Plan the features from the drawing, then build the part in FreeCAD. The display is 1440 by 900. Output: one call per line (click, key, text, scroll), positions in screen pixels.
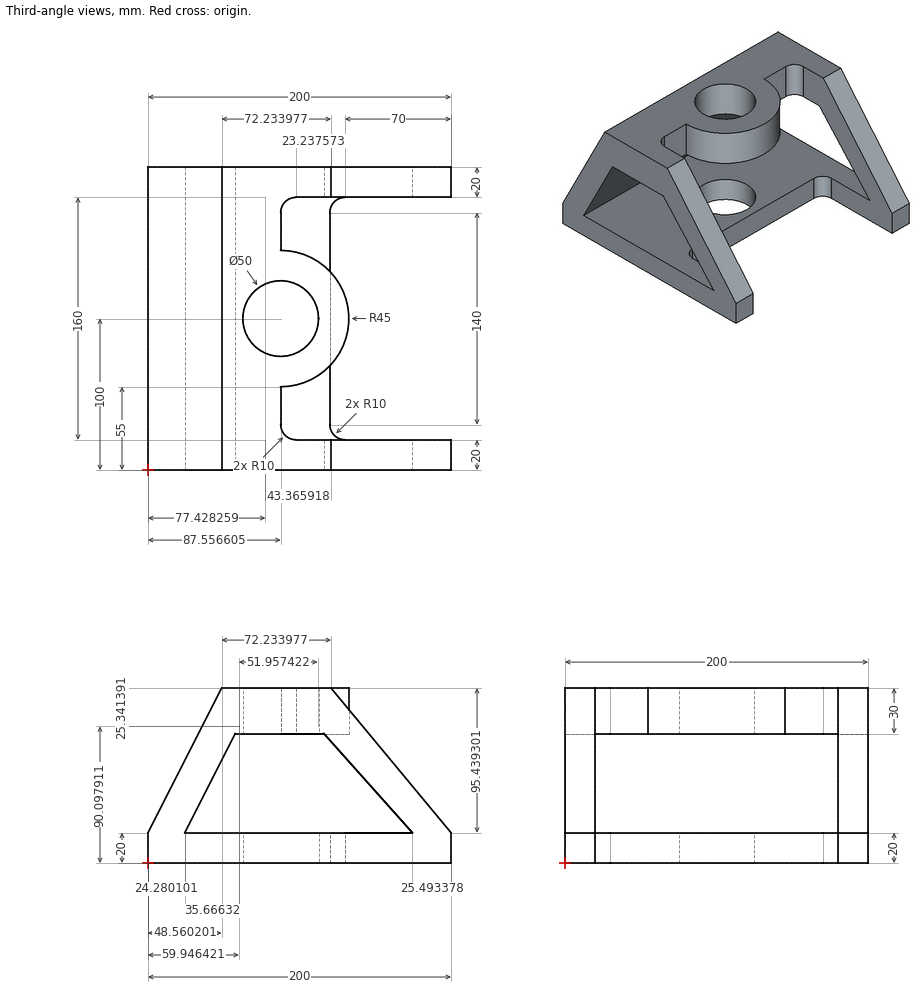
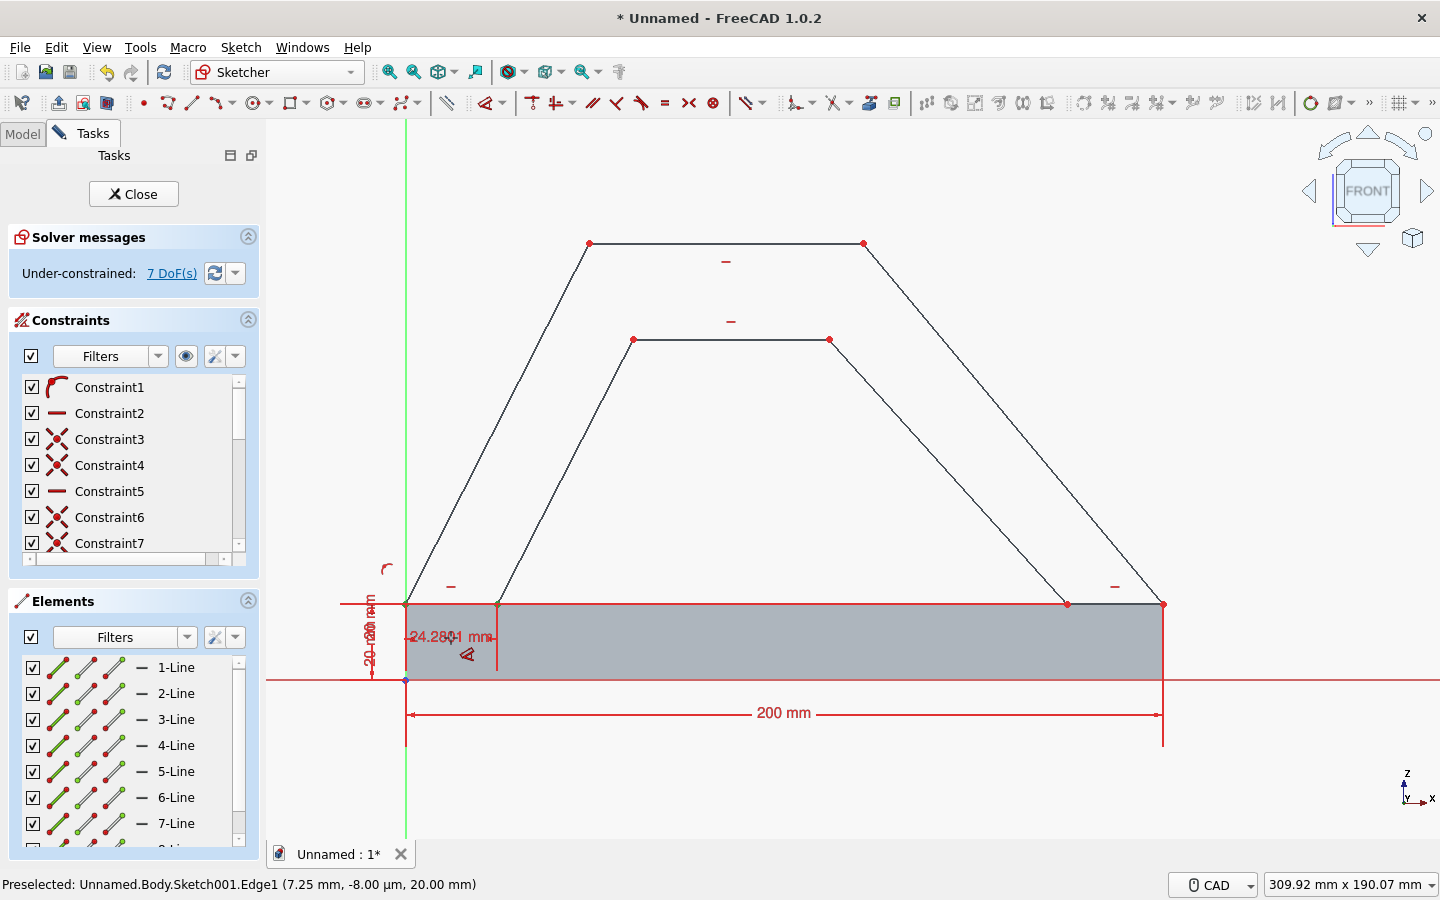
click(692, 340)
click(731, 306)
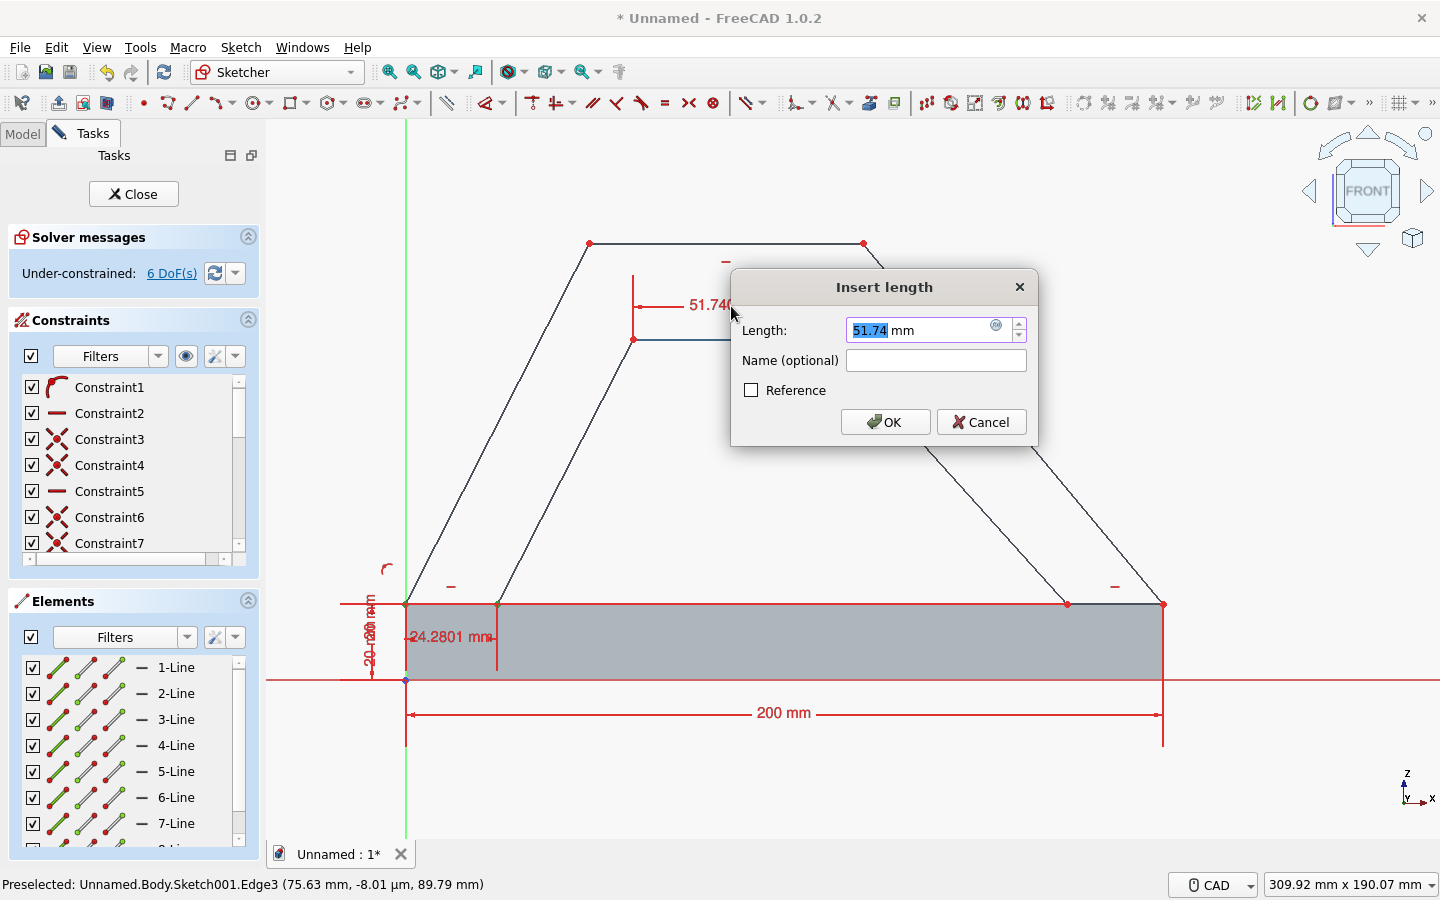
text(51.957422)
key(Return)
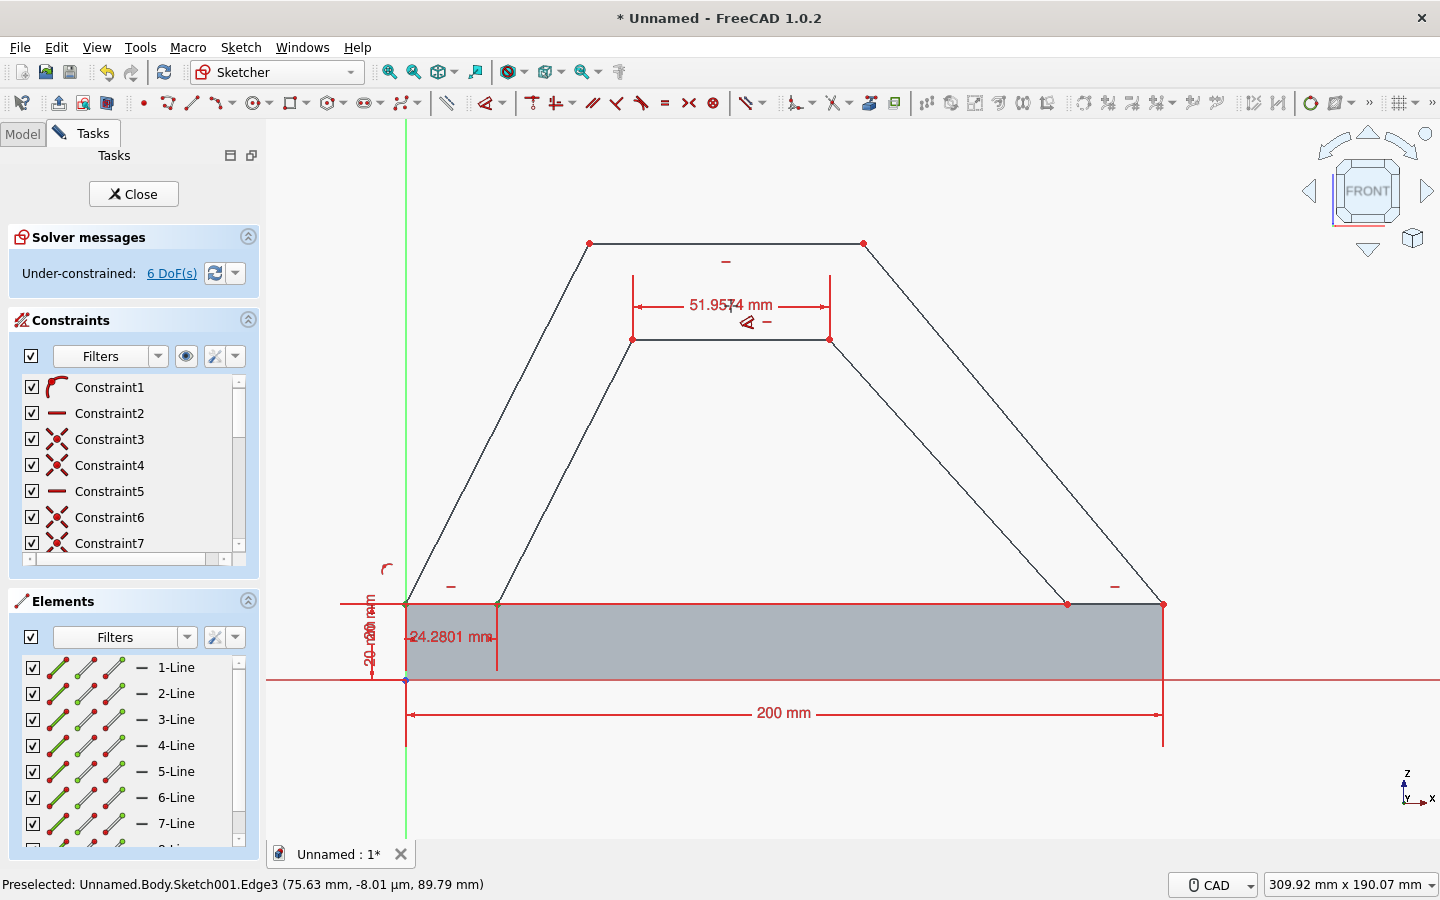
click(1096, 604)
click(1115, 638)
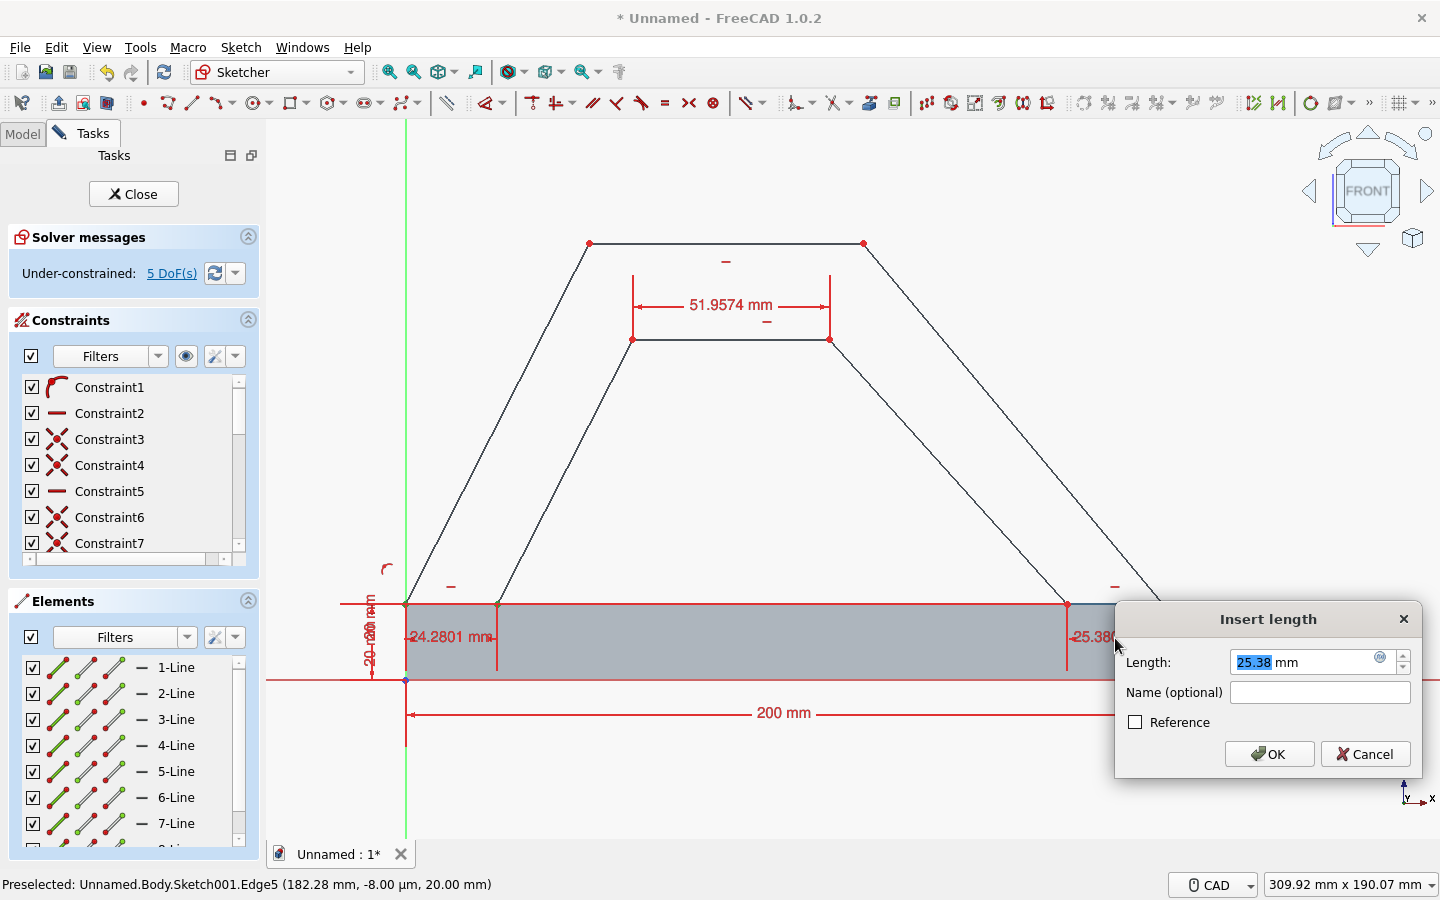
text(25.493378)
key(Return)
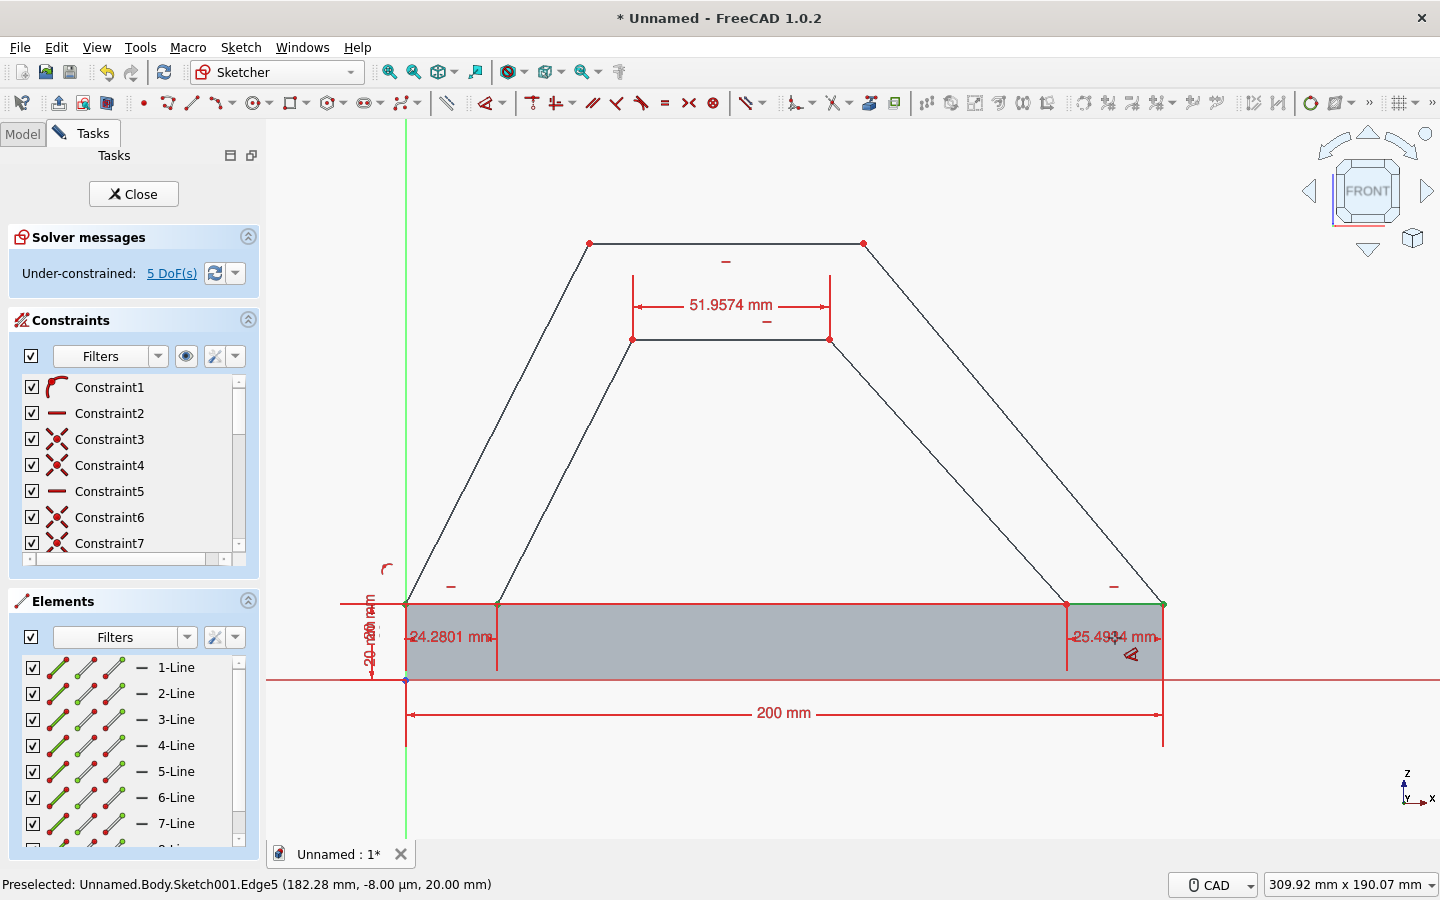
click(781, 244)
click(726, 210)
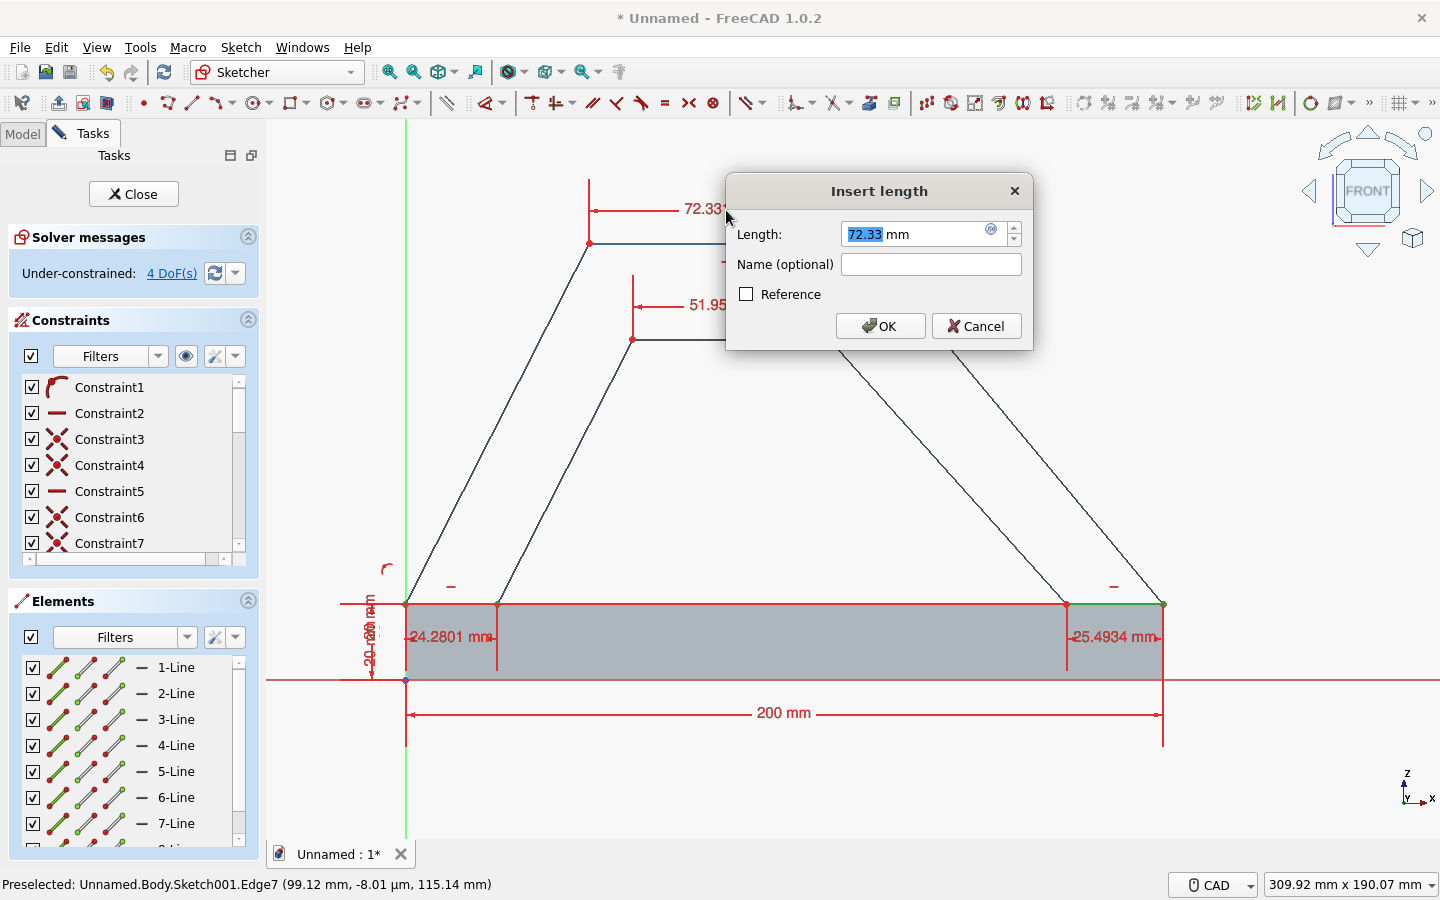
text(72.233977)
key(Return)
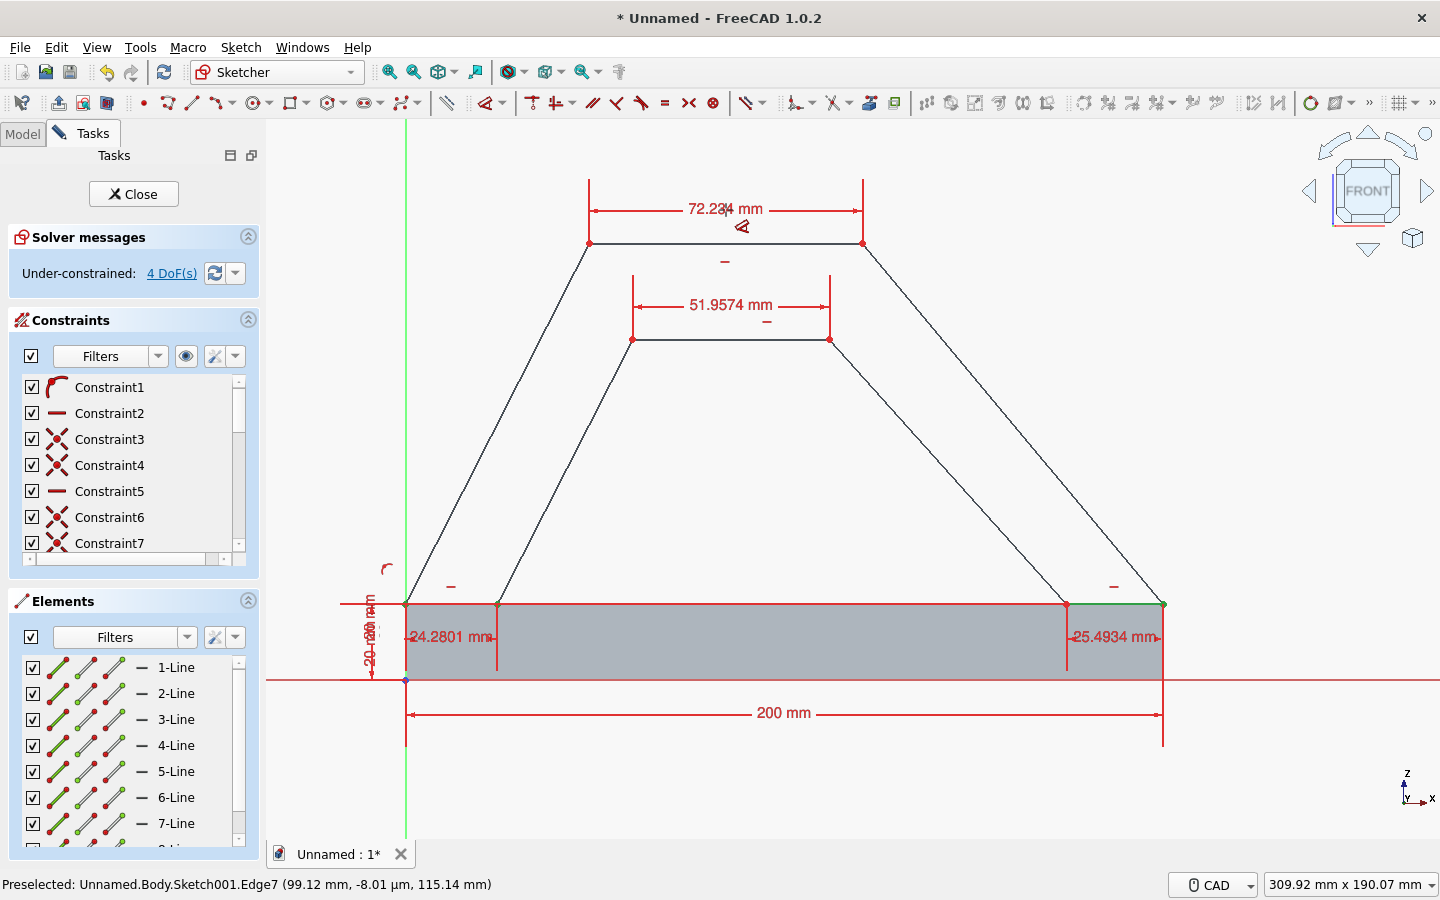
click(538, 525)
click(565, 638)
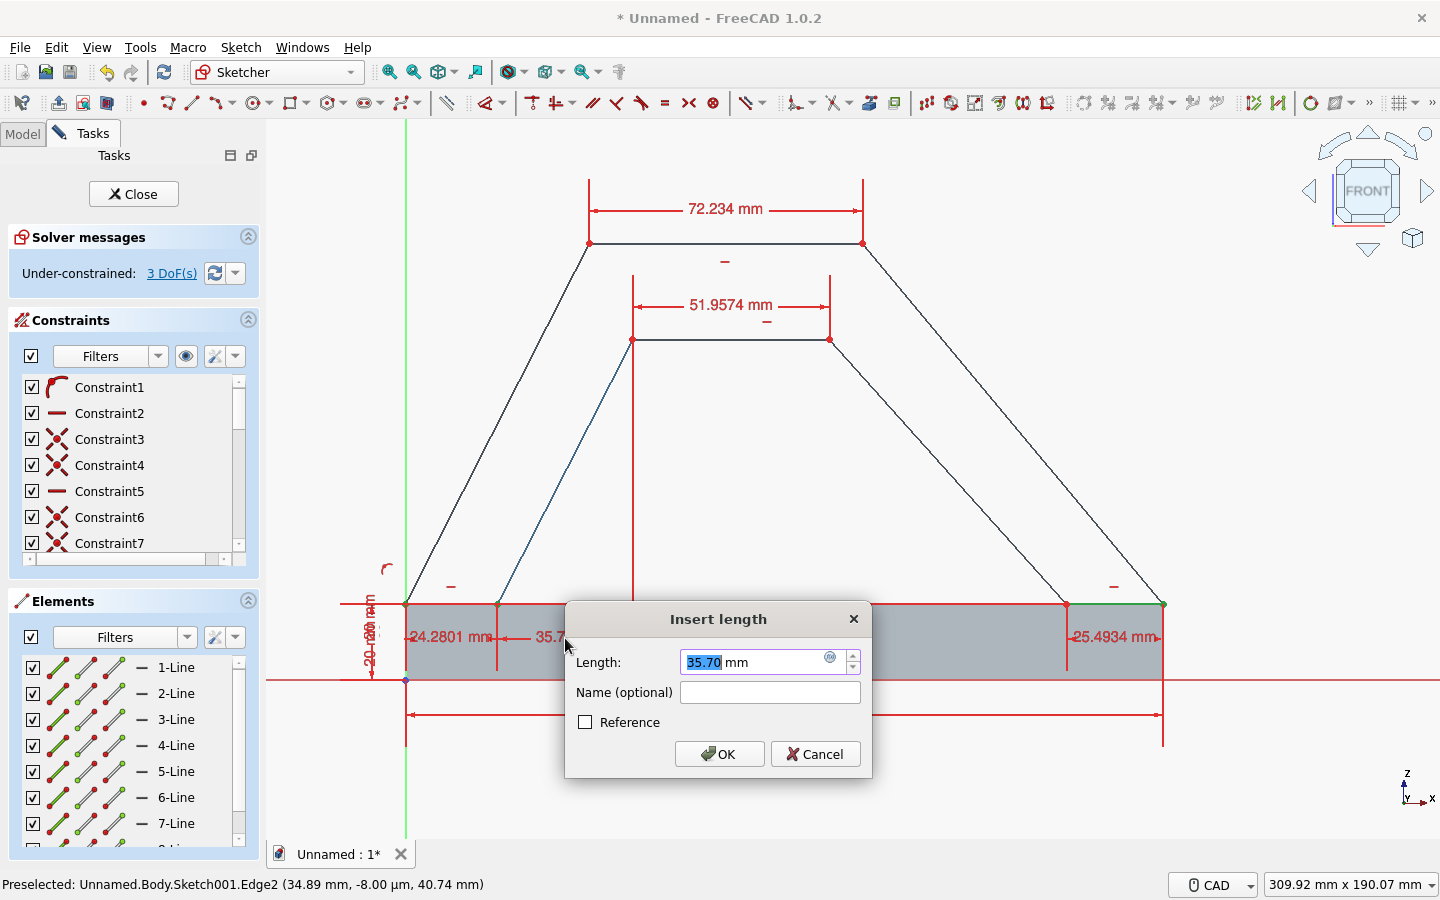
text(35.66632)
key(Return)